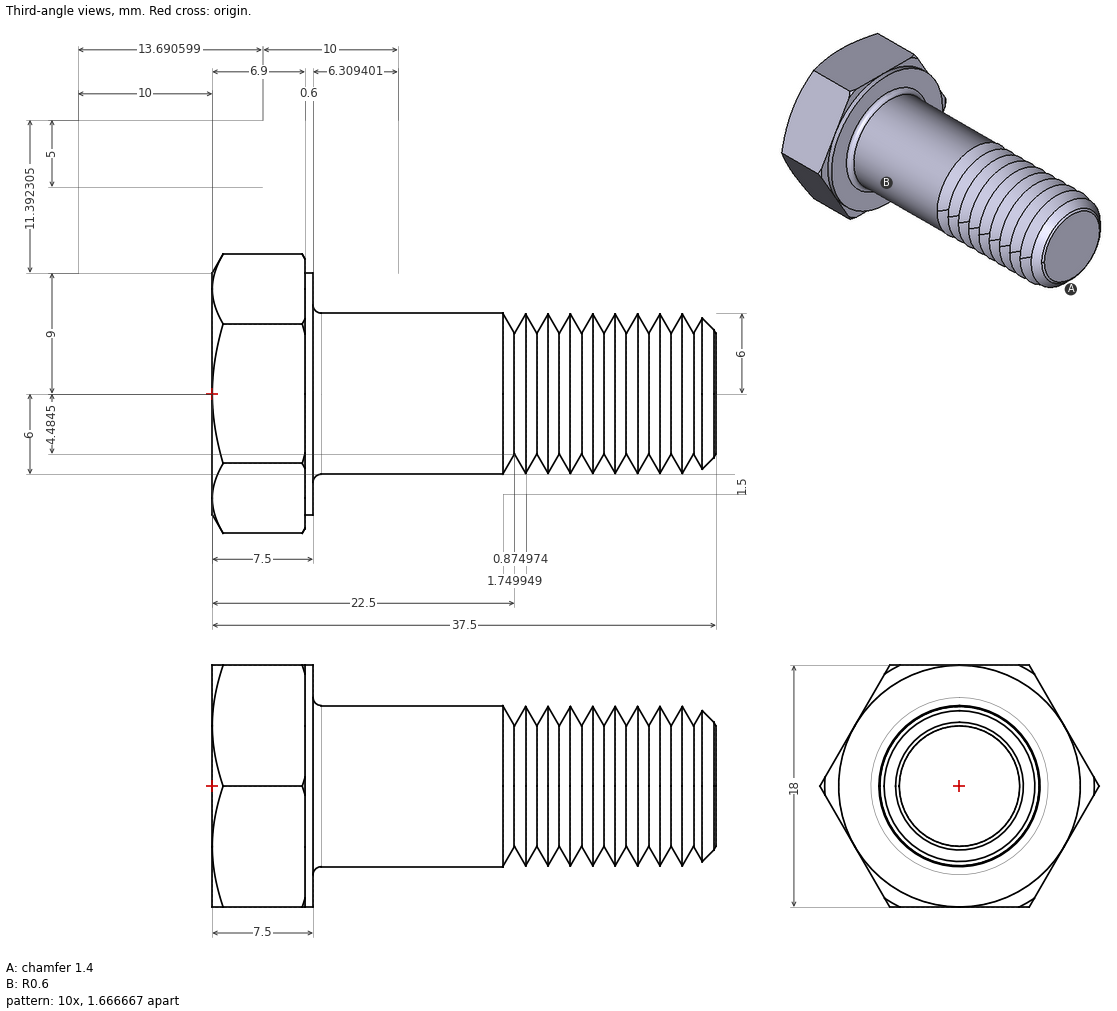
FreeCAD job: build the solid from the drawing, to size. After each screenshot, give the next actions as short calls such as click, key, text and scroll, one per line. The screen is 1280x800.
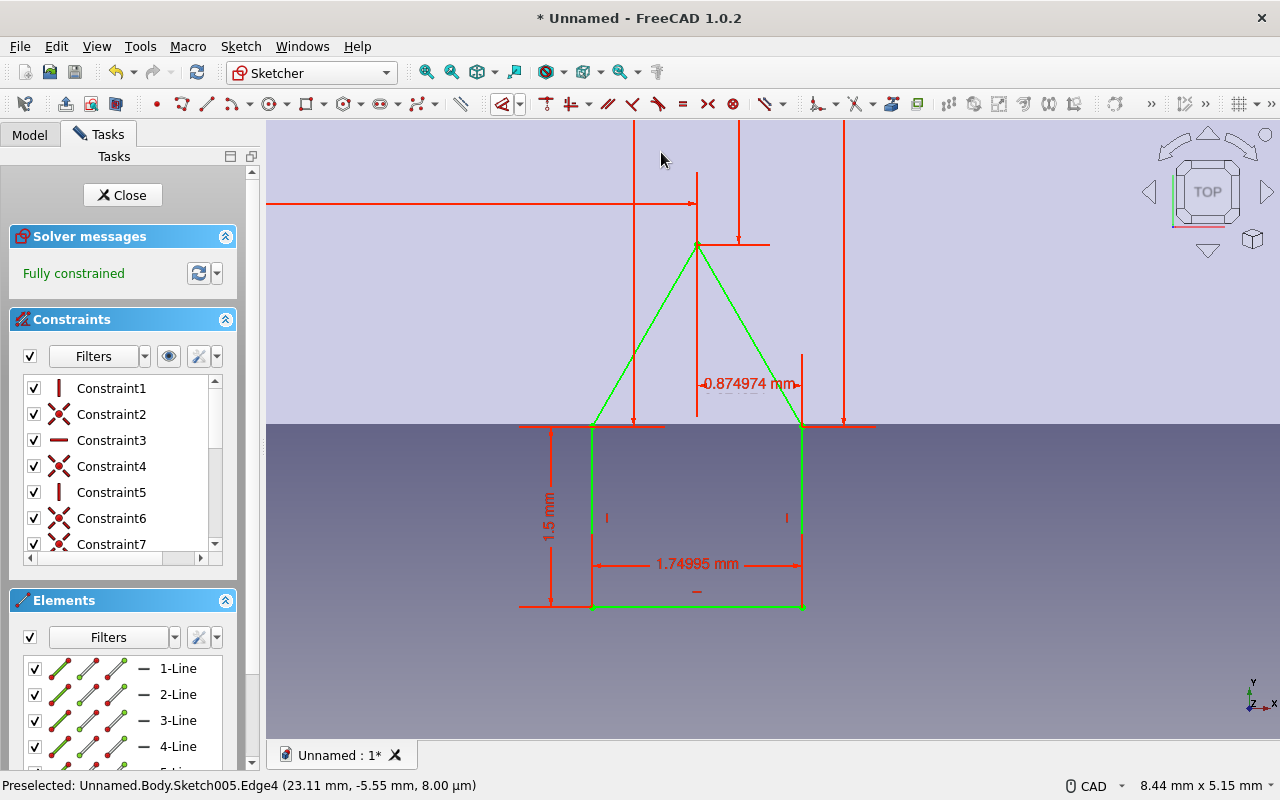
click(123, 195)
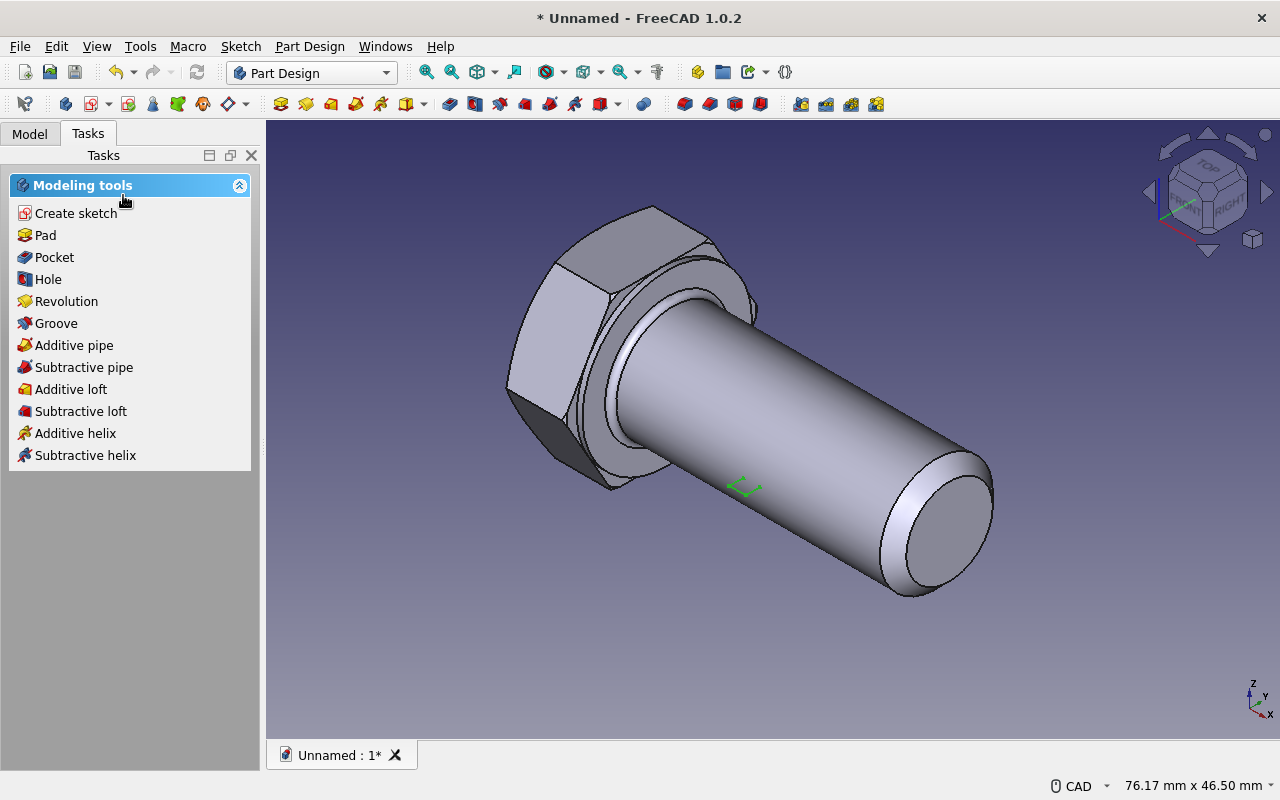
click(500, 104)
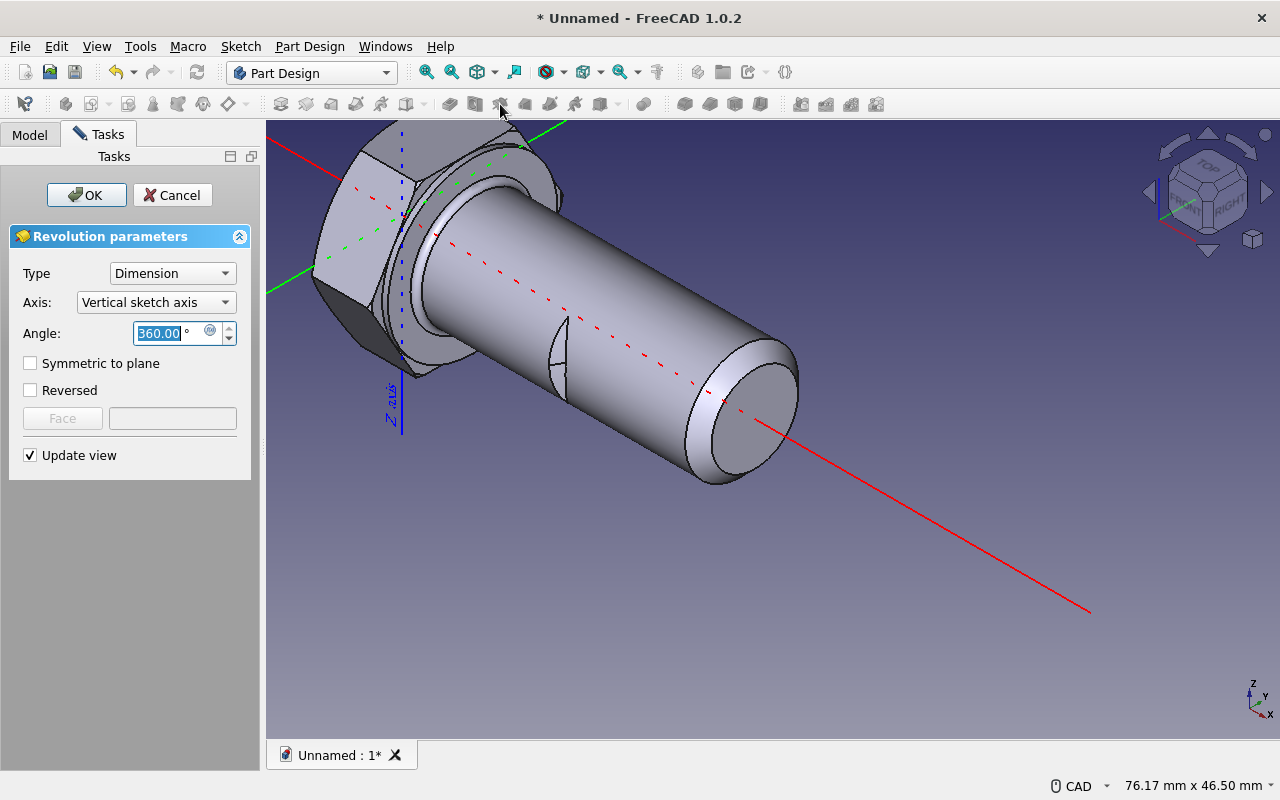
click(157, 302)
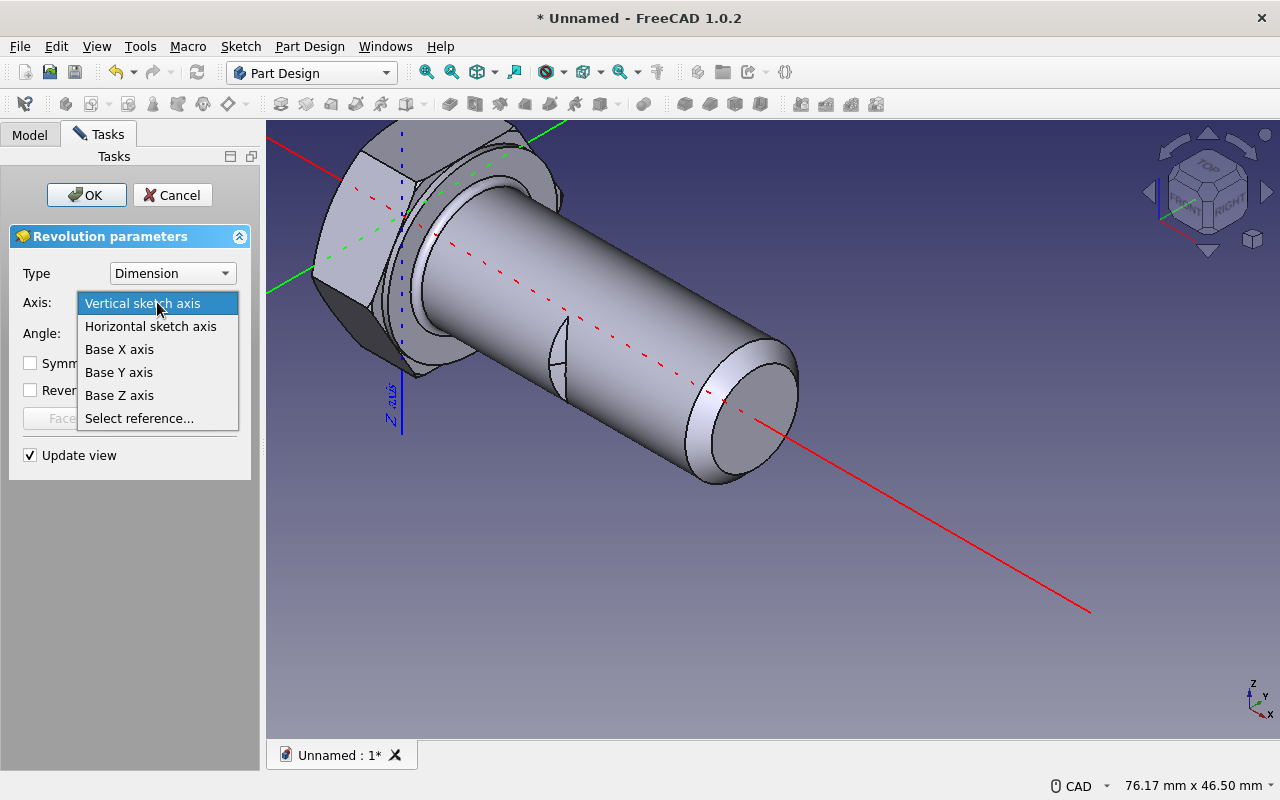
click(156, 326)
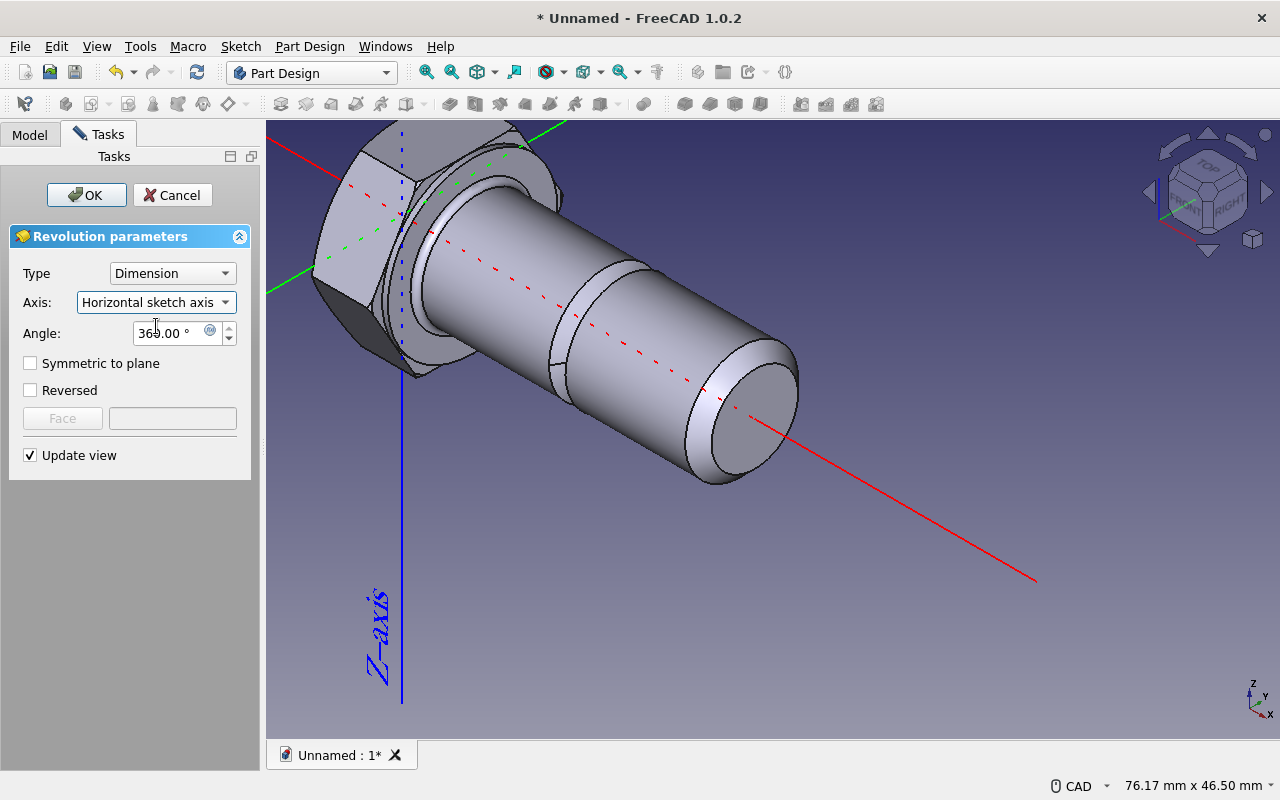
click(87, 195)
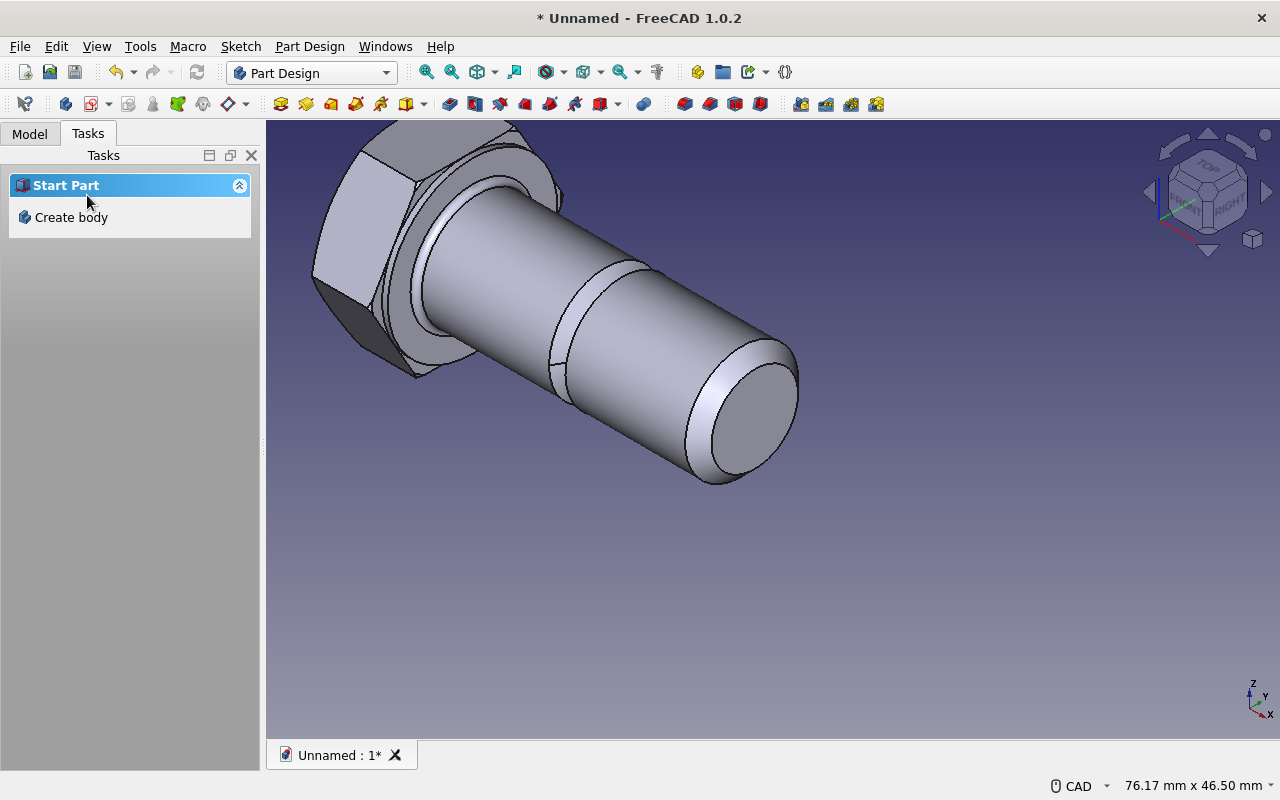
click(427, 72)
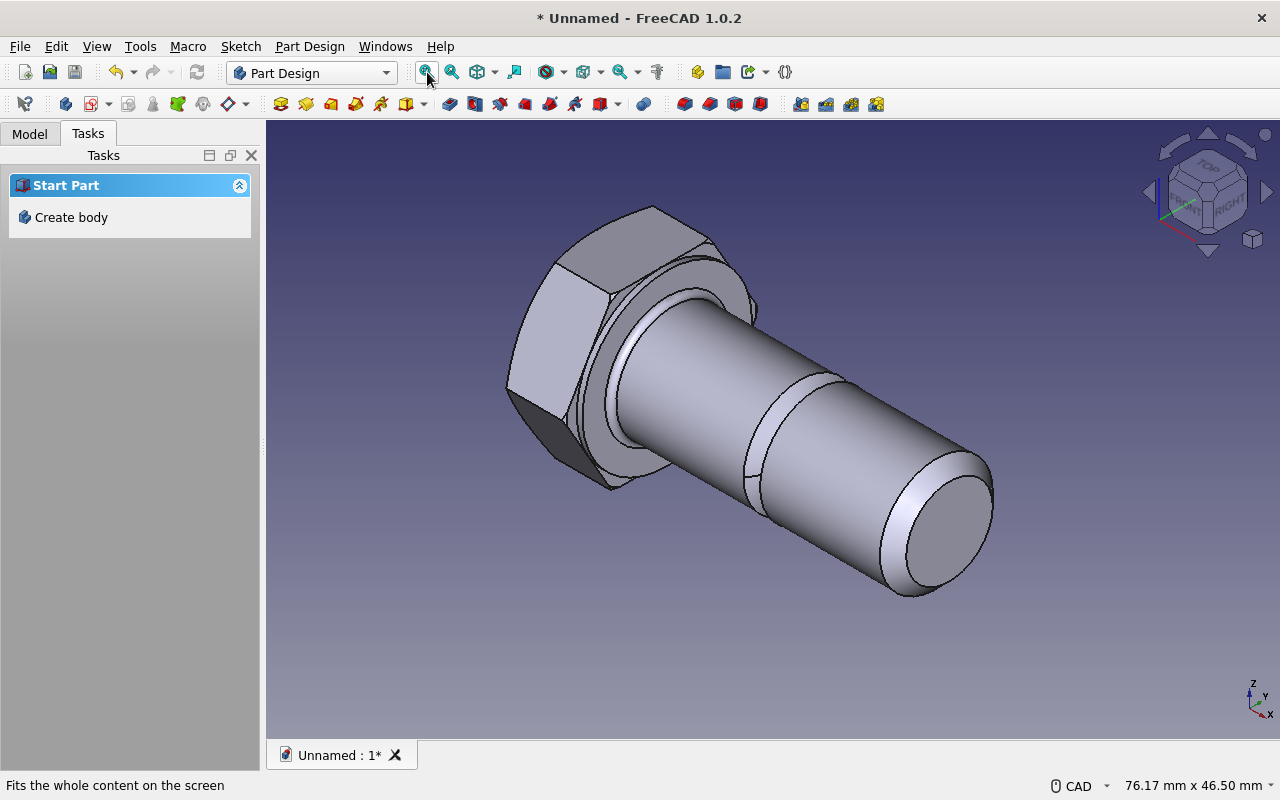
click(30, 134)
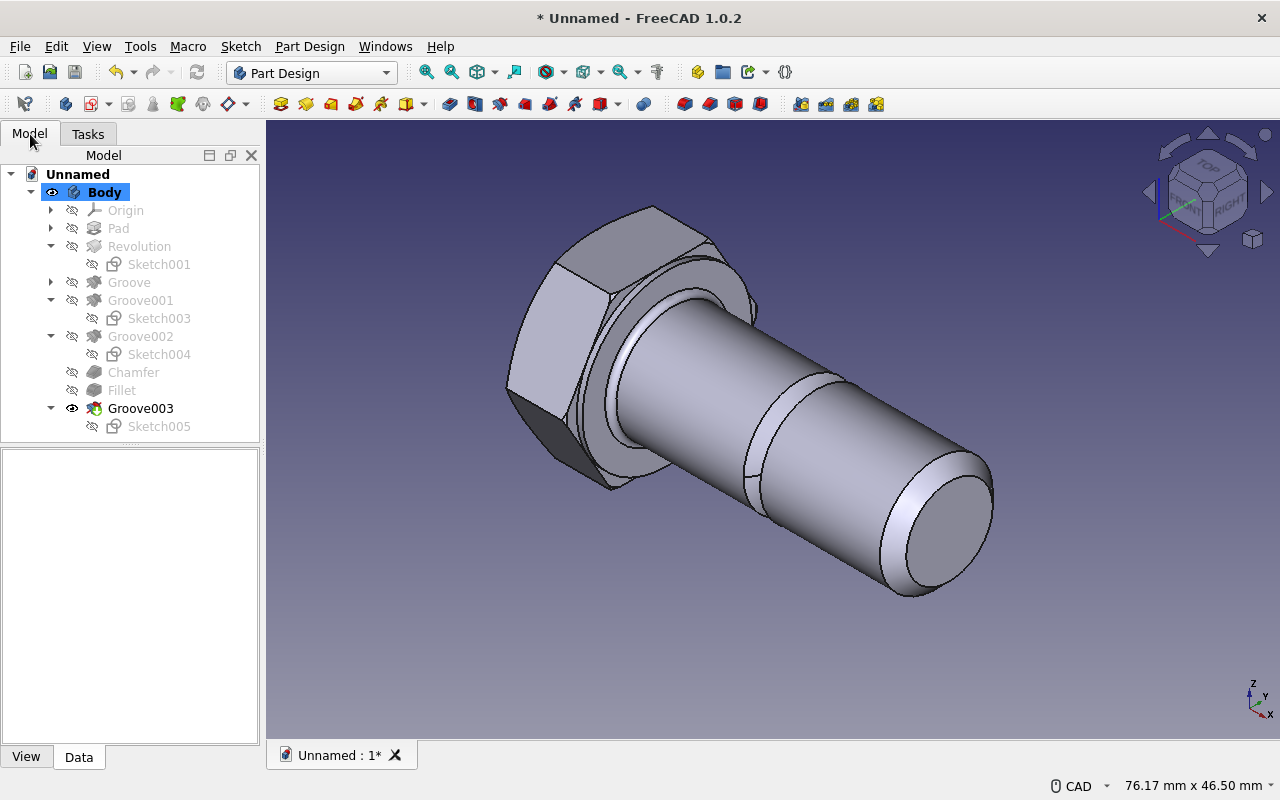
click(117, 408)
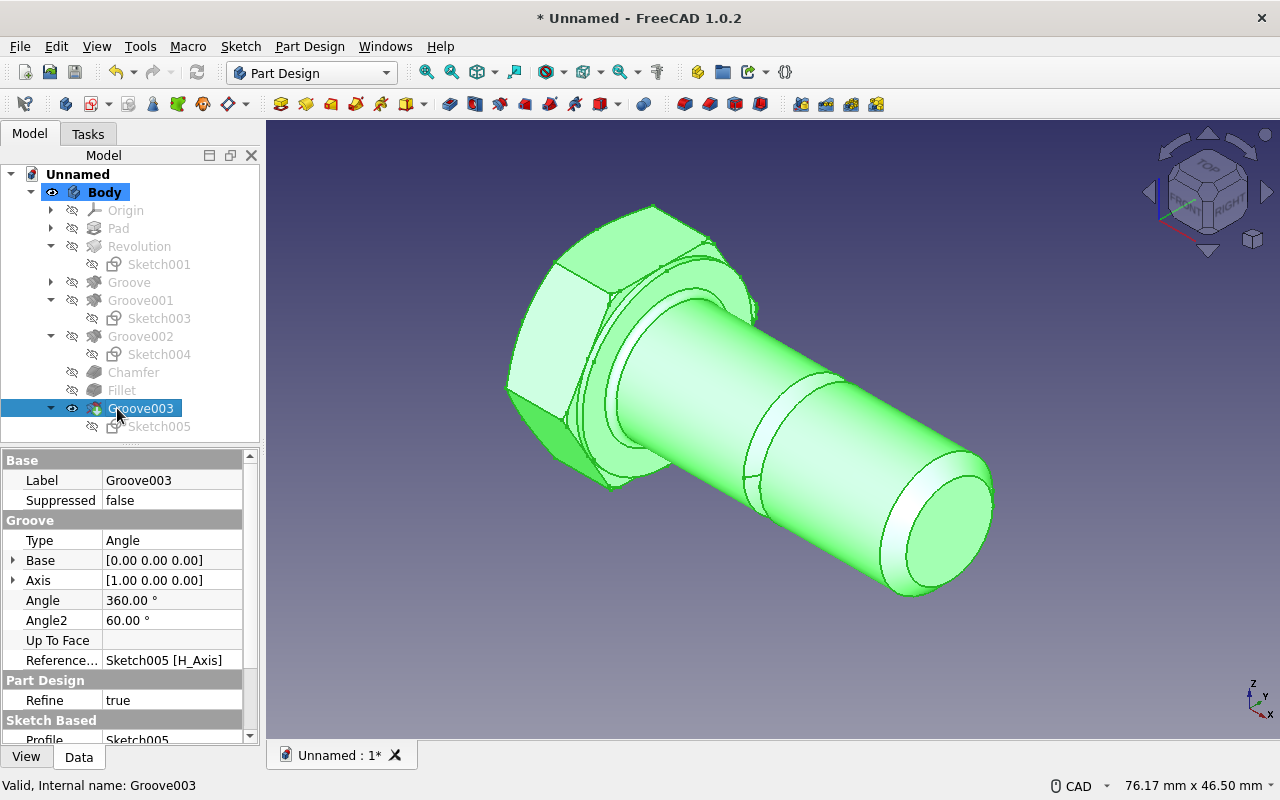
click(826, 104)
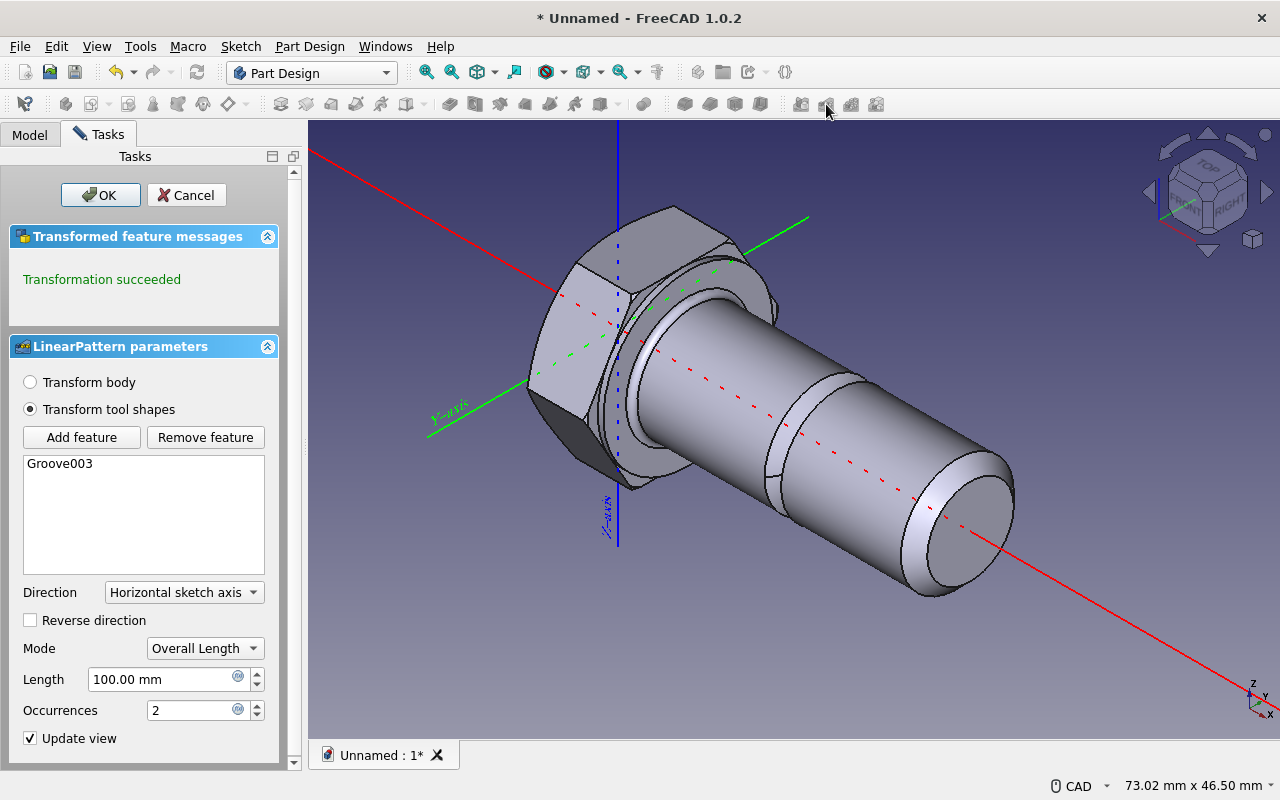
click(185, 592)